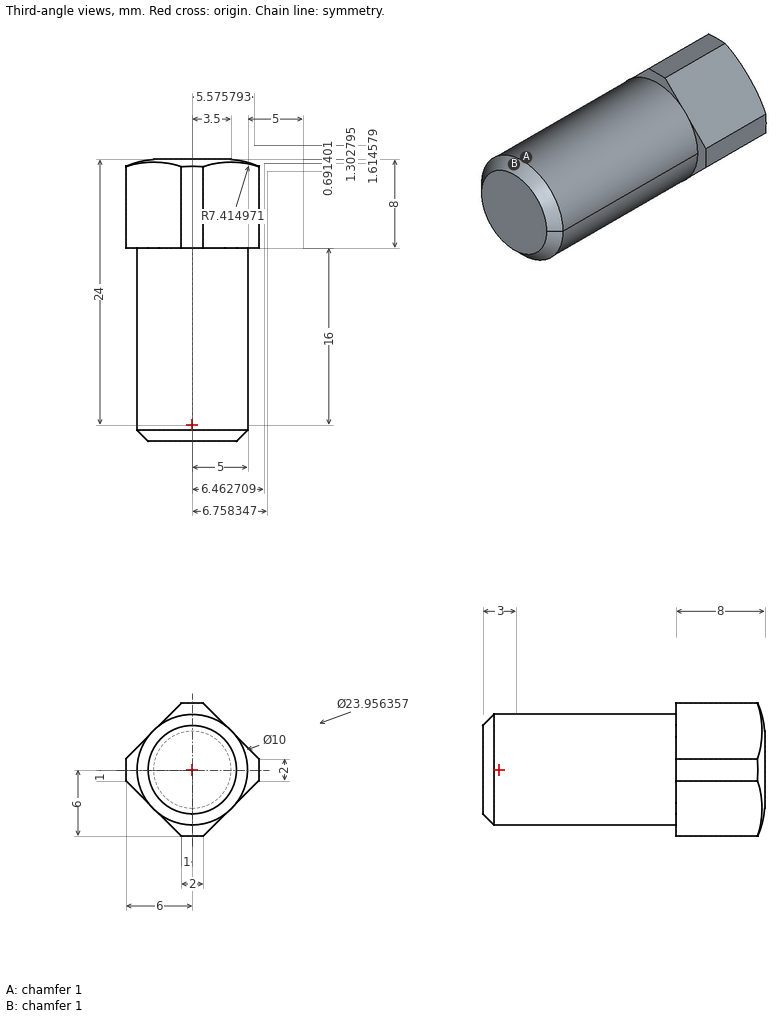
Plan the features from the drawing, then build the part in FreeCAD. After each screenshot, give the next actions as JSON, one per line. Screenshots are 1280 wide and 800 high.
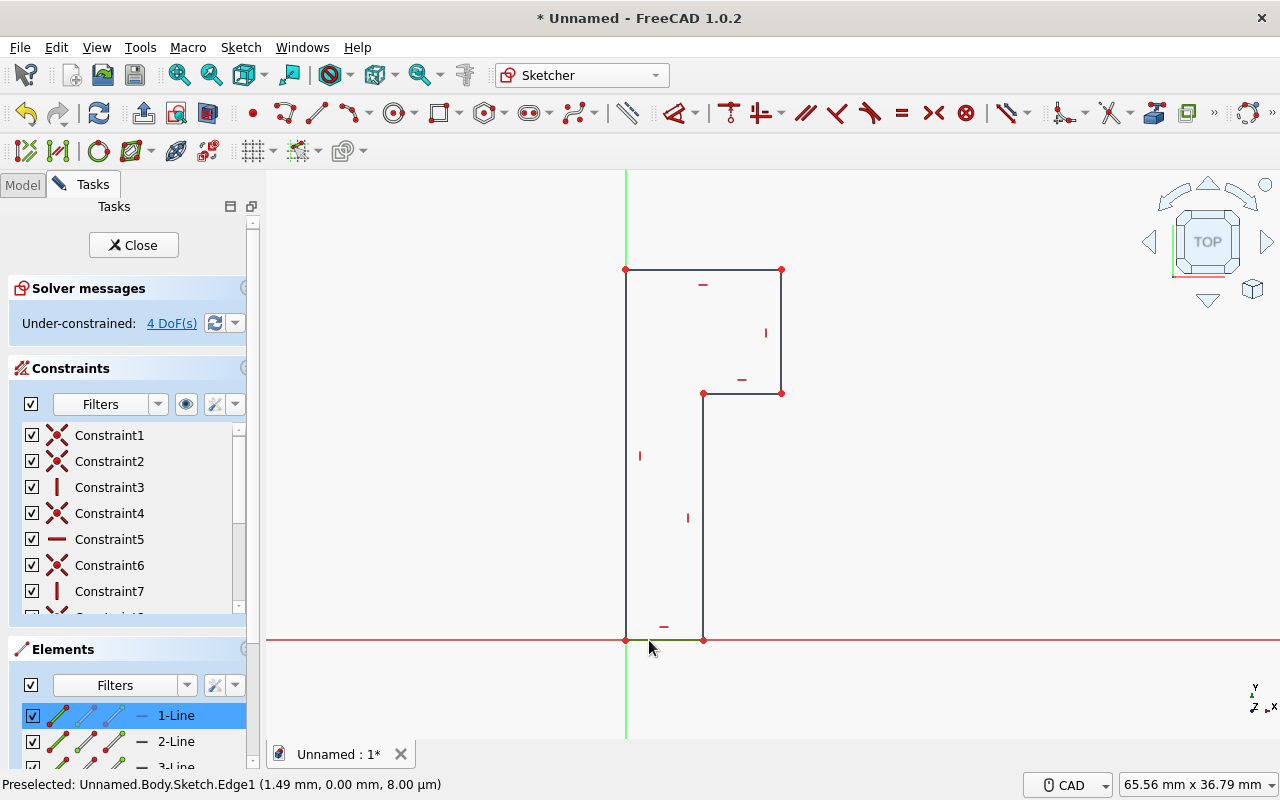
{"action": "left_click", "coordinate": [698, 114]}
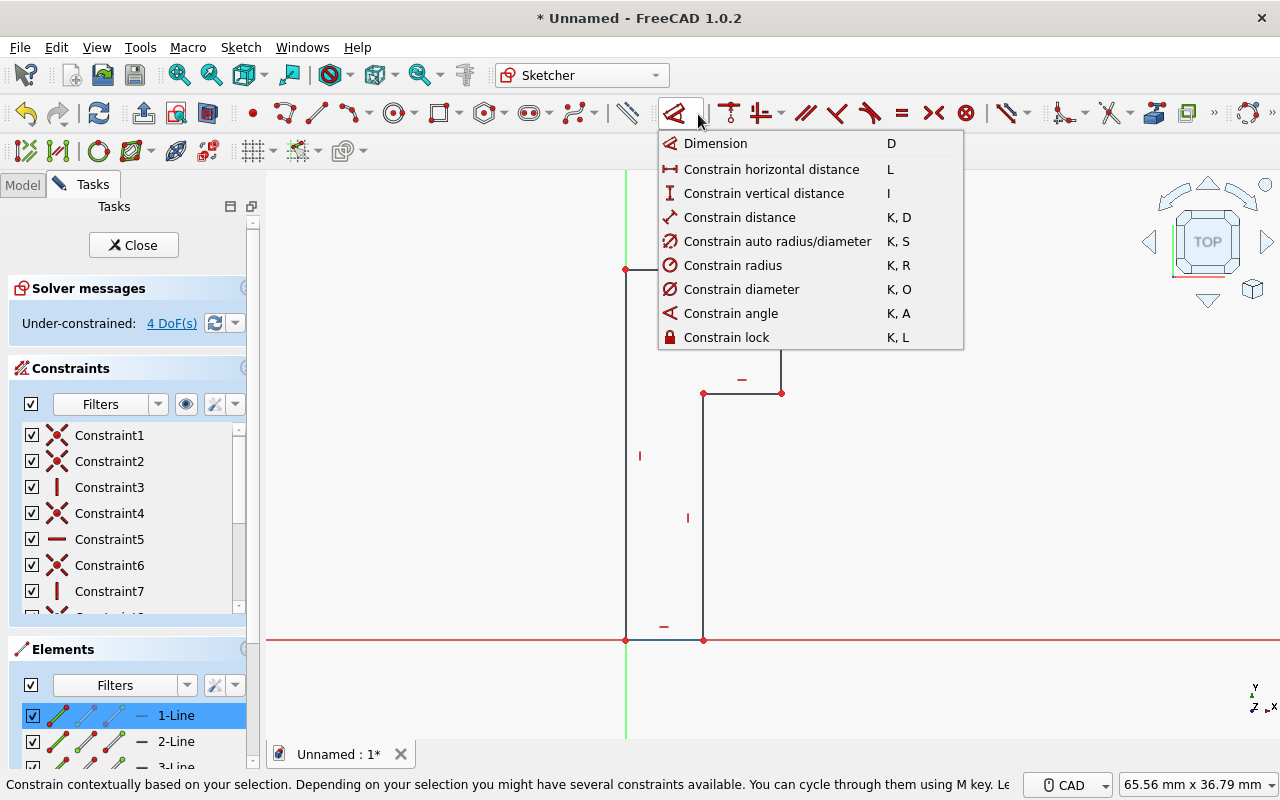
{"action": "left_click", "coordinate": [811, 169]}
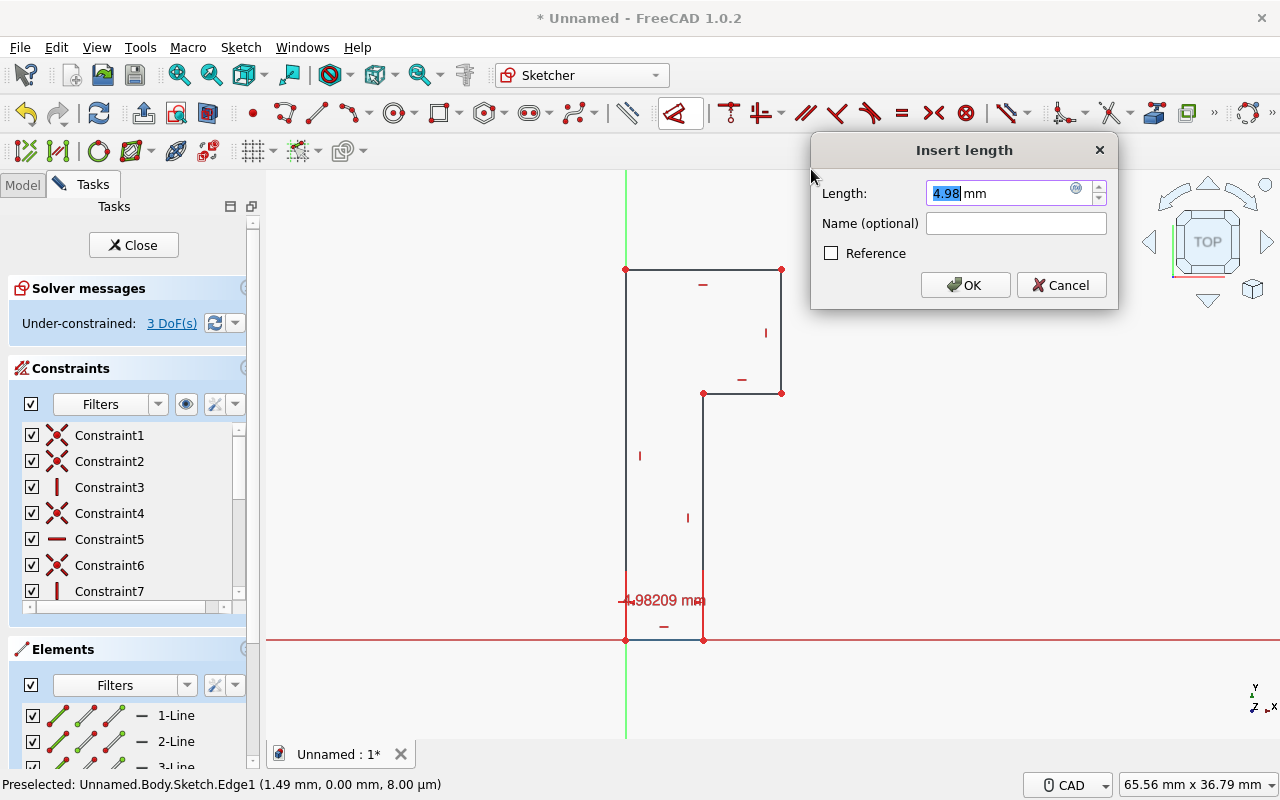
{"action": "type", "text": "5"}
{"action": "key", "text": "Return"}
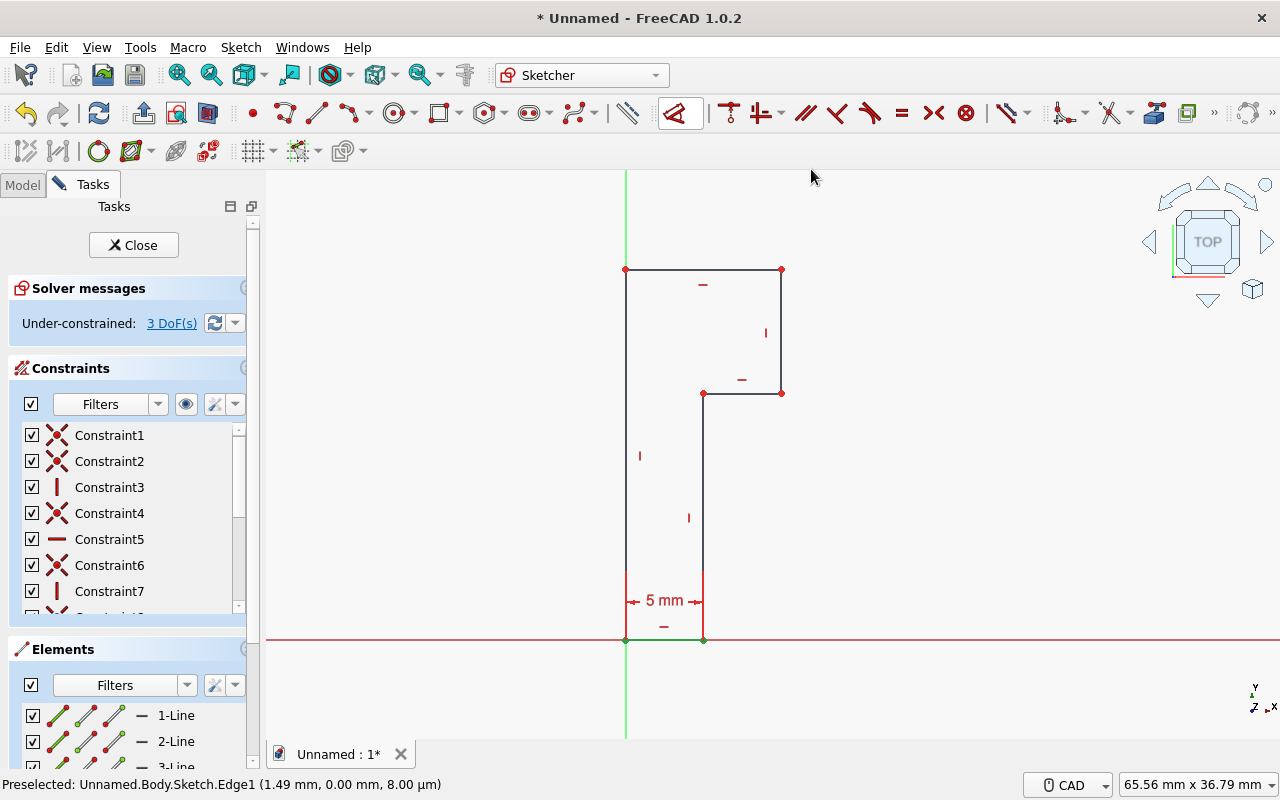
{"action": "left_click", "coordinate": [727, 394]}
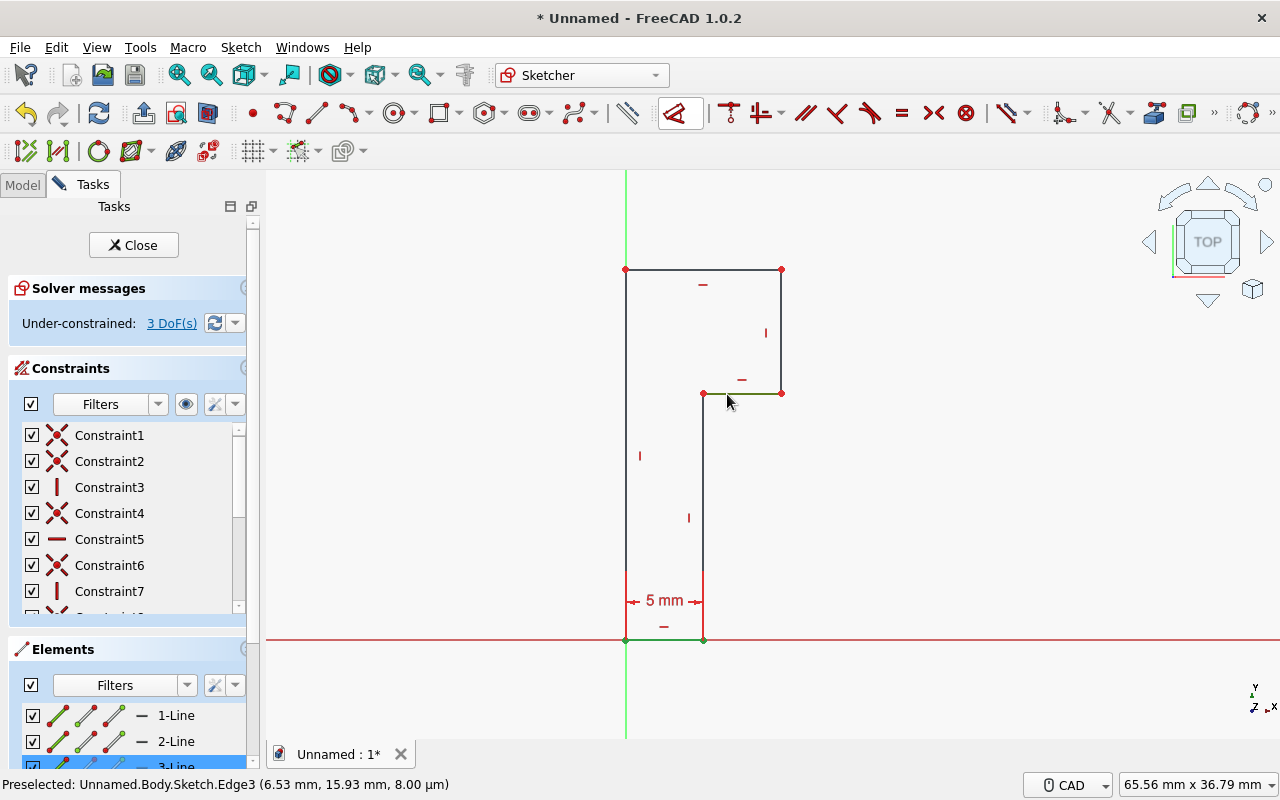
{"action": "key", "text": "l"}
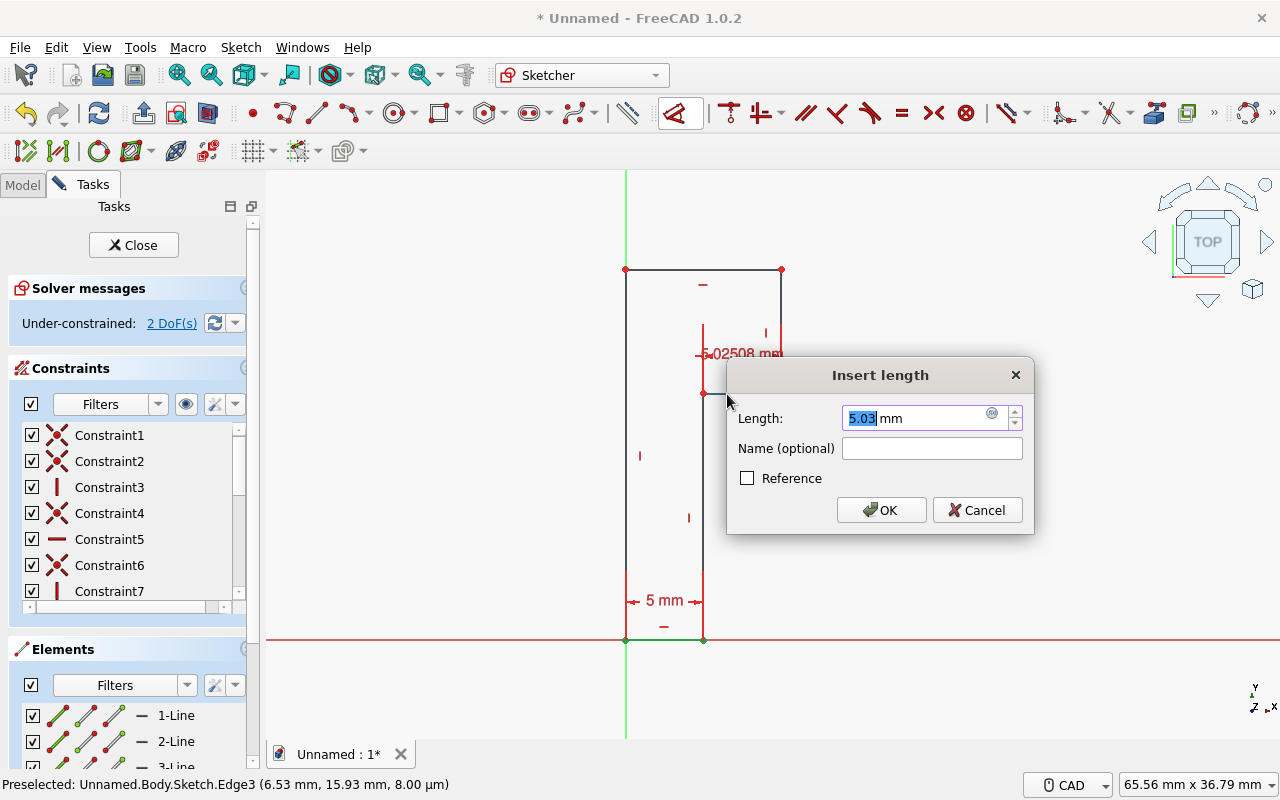
{"action": "type", "text": "5"}
{"action": "key", "text": "Return"}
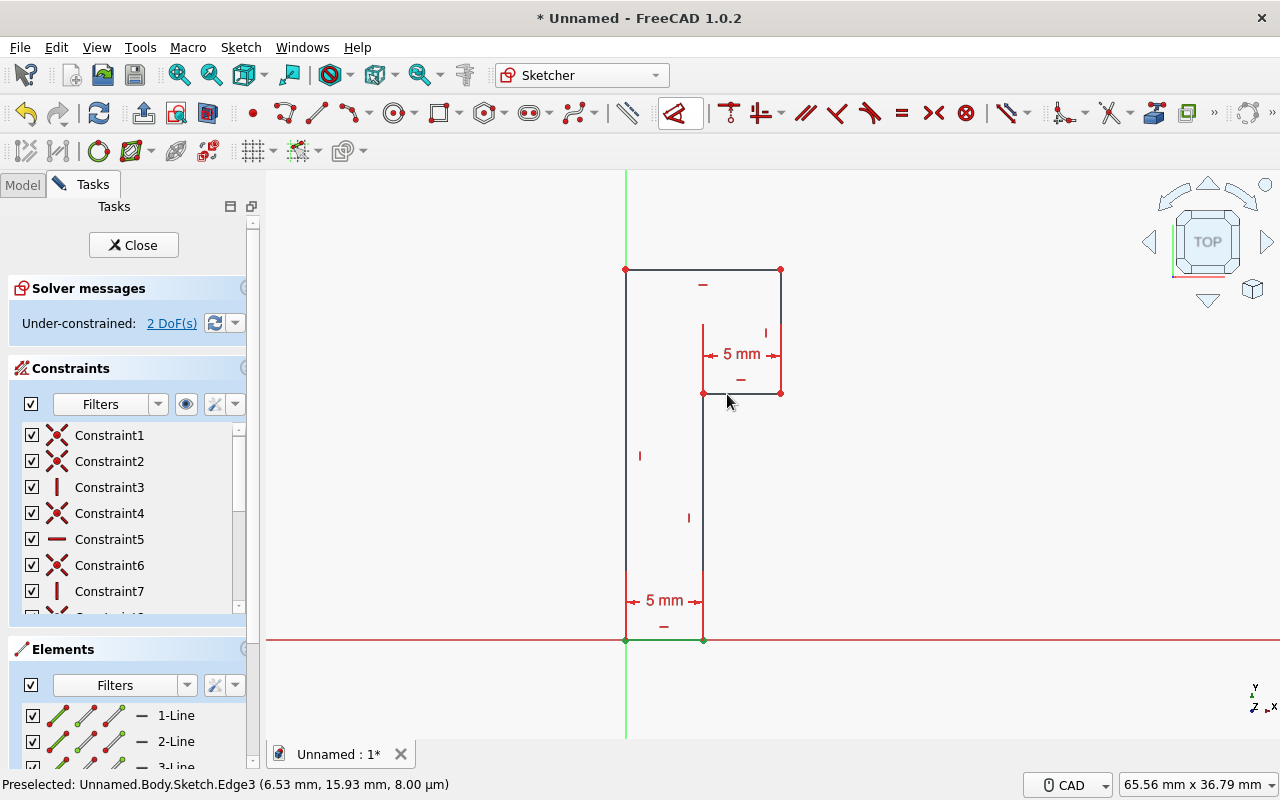
{"action": "left_click", "coordinate": [781, 357]}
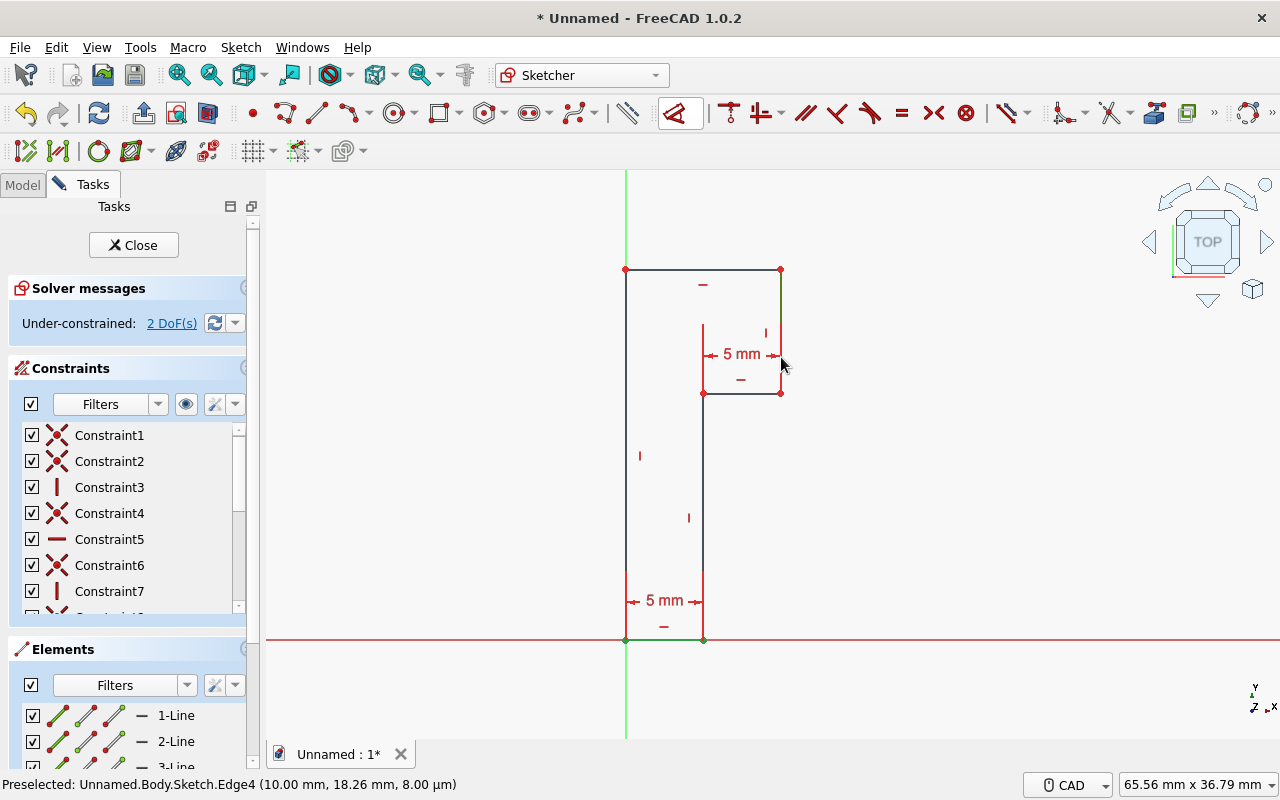
{"action": "key", "text": "i"}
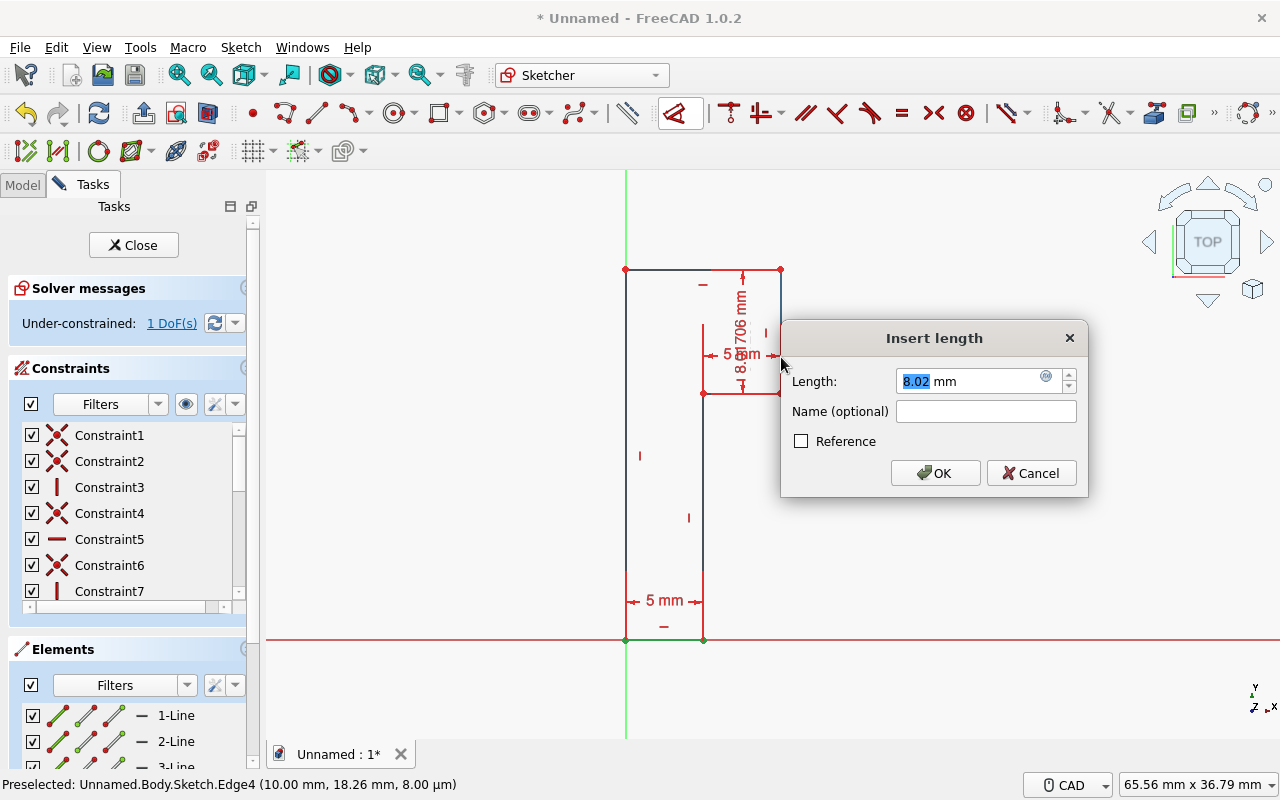
{"action": "type", "text": "8"}
{"action": "key", "text": "Return"}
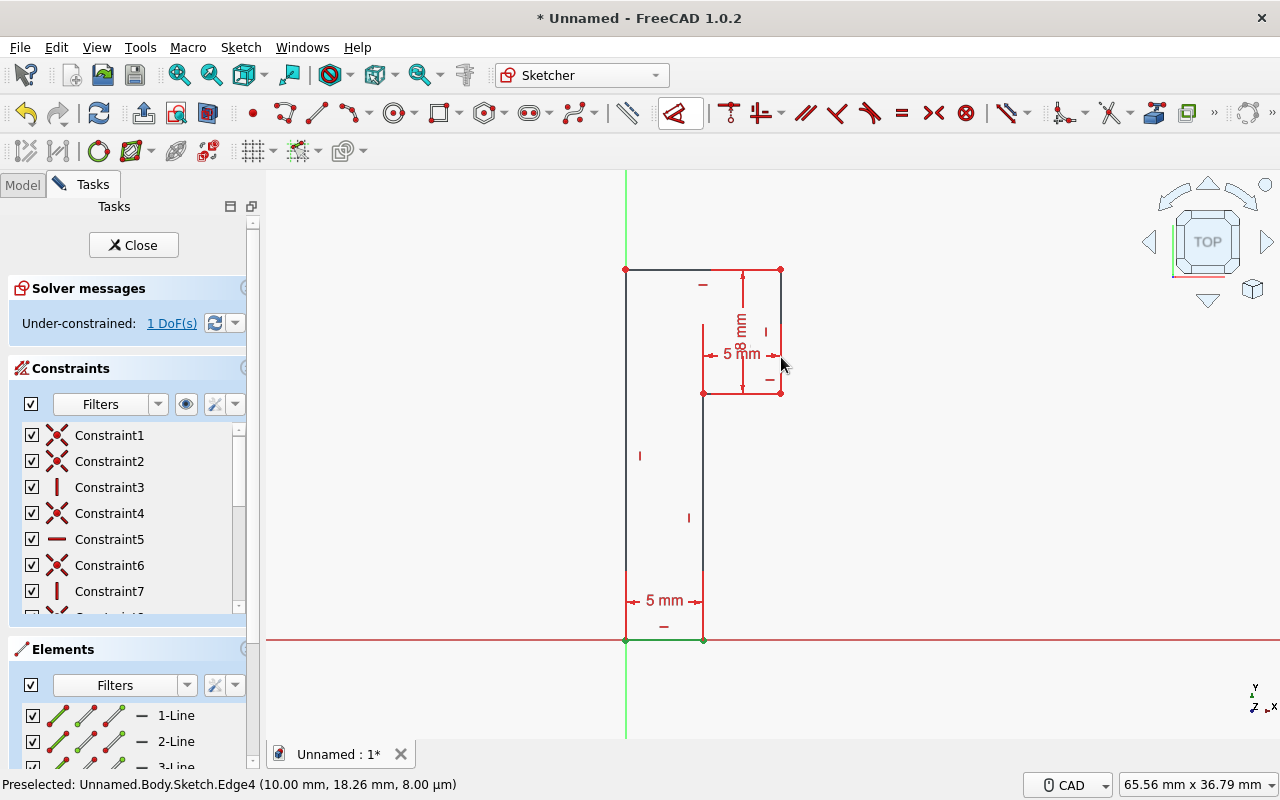
{"action": "left_click", "coordinate": [703, 566]}